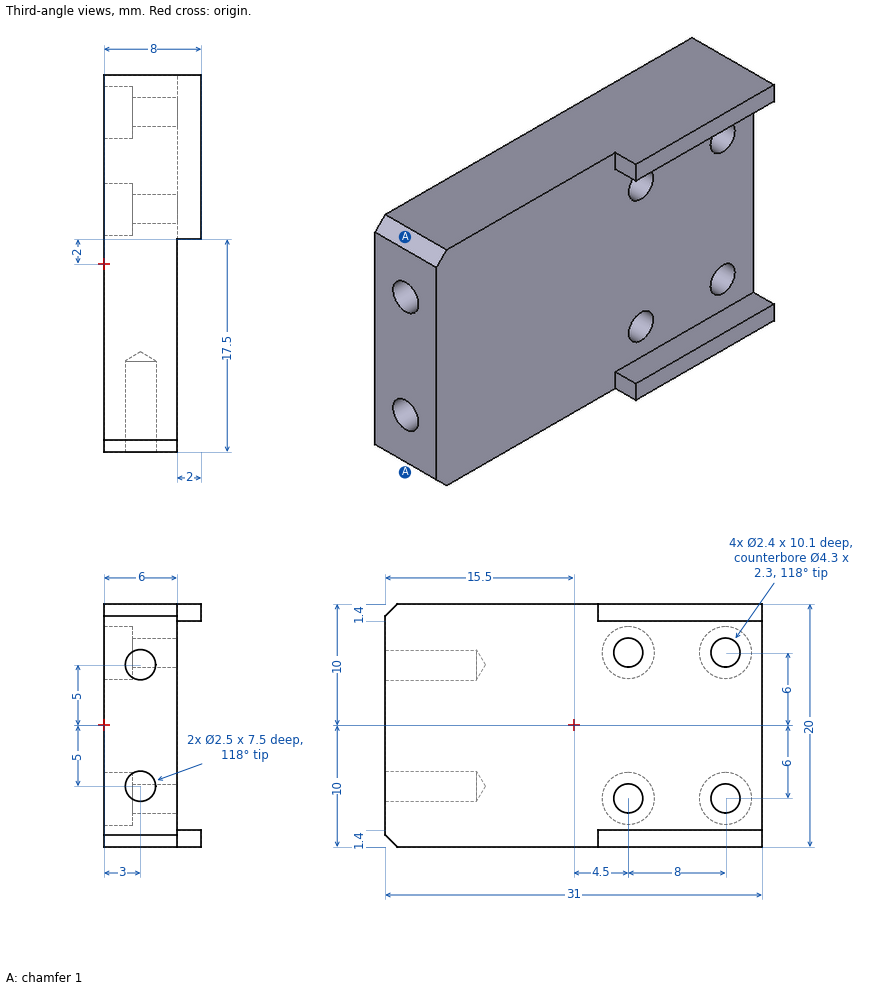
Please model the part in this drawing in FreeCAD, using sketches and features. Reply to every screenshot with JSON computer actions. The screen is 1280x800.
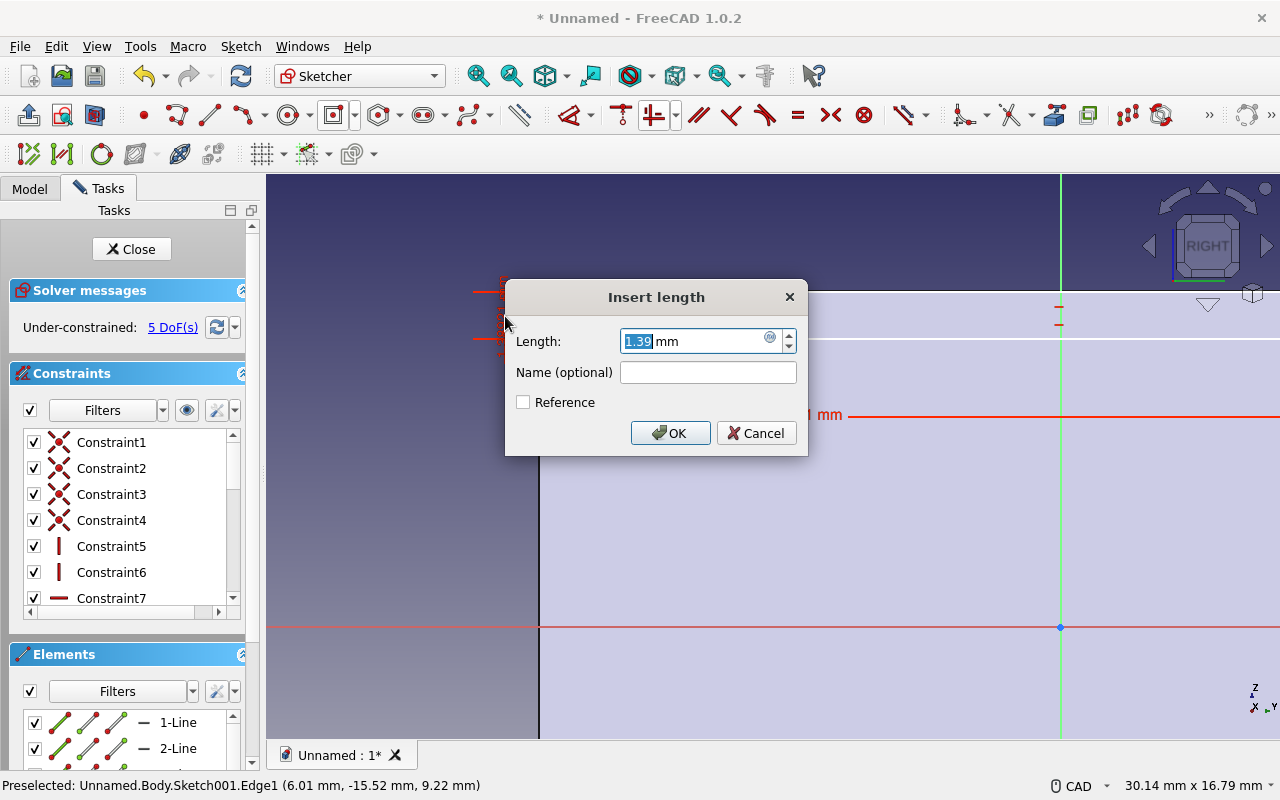
{"action": "type", "text": "1.4"}
{"action": "key", "text": "Return"}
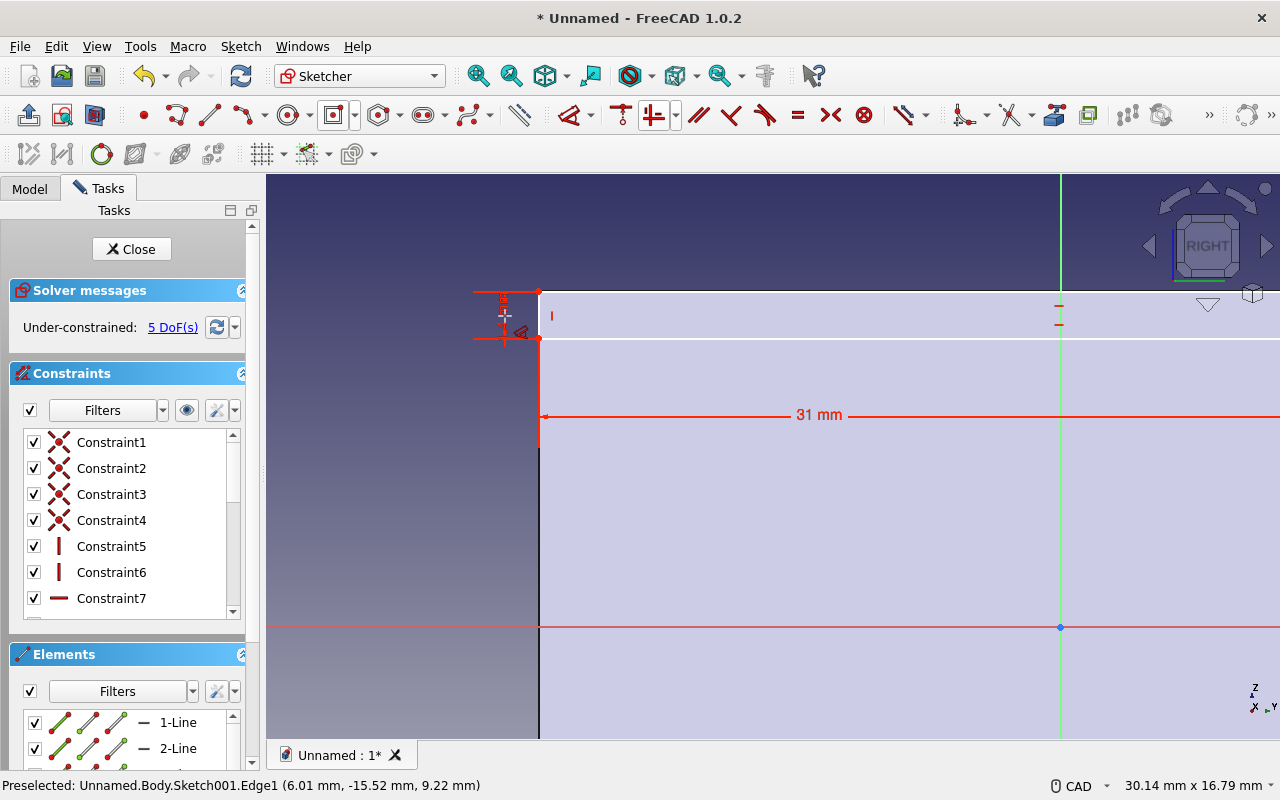
{"action": "scroll", "coordinate": [294, 249], "scroll_direction": "down", "scroll_amount": 3}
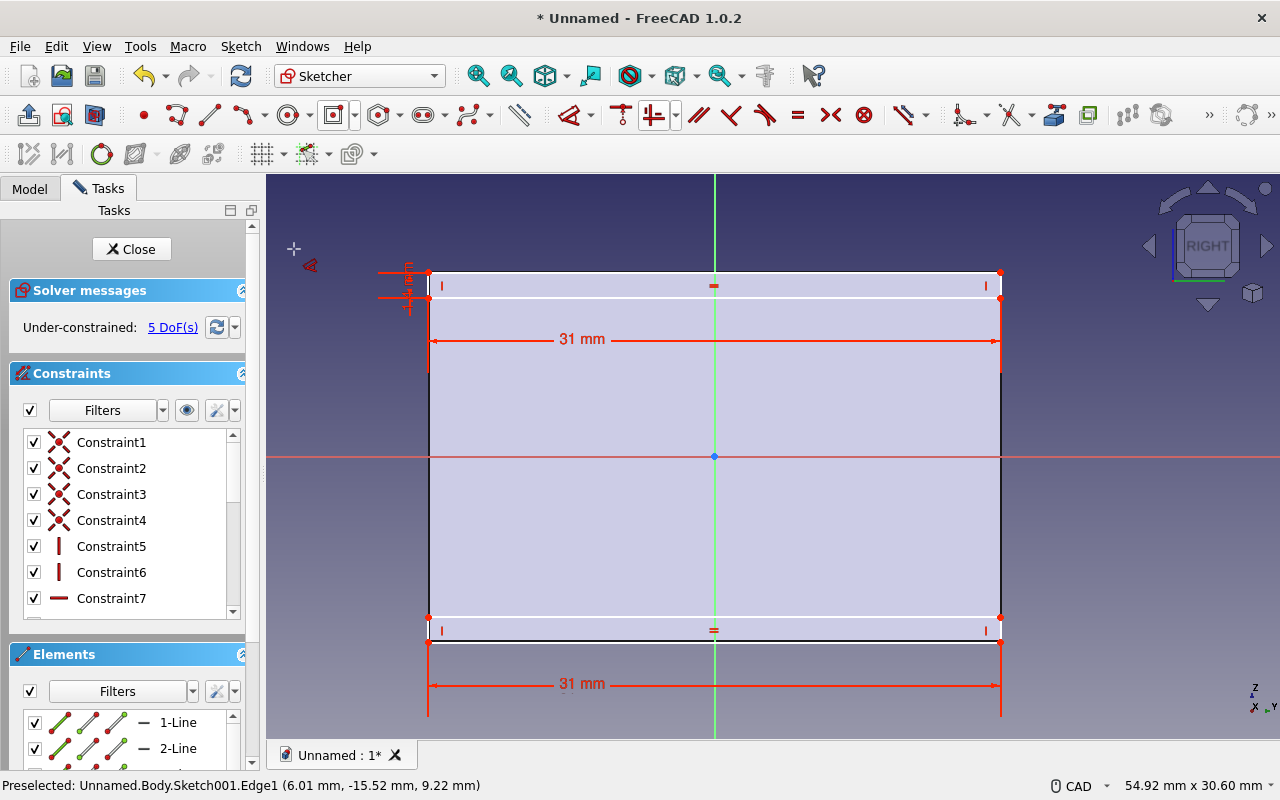
{"action": "scroll", "coordinate": [428, 625], "scroll_direction": "up", "scroll_amount": 3}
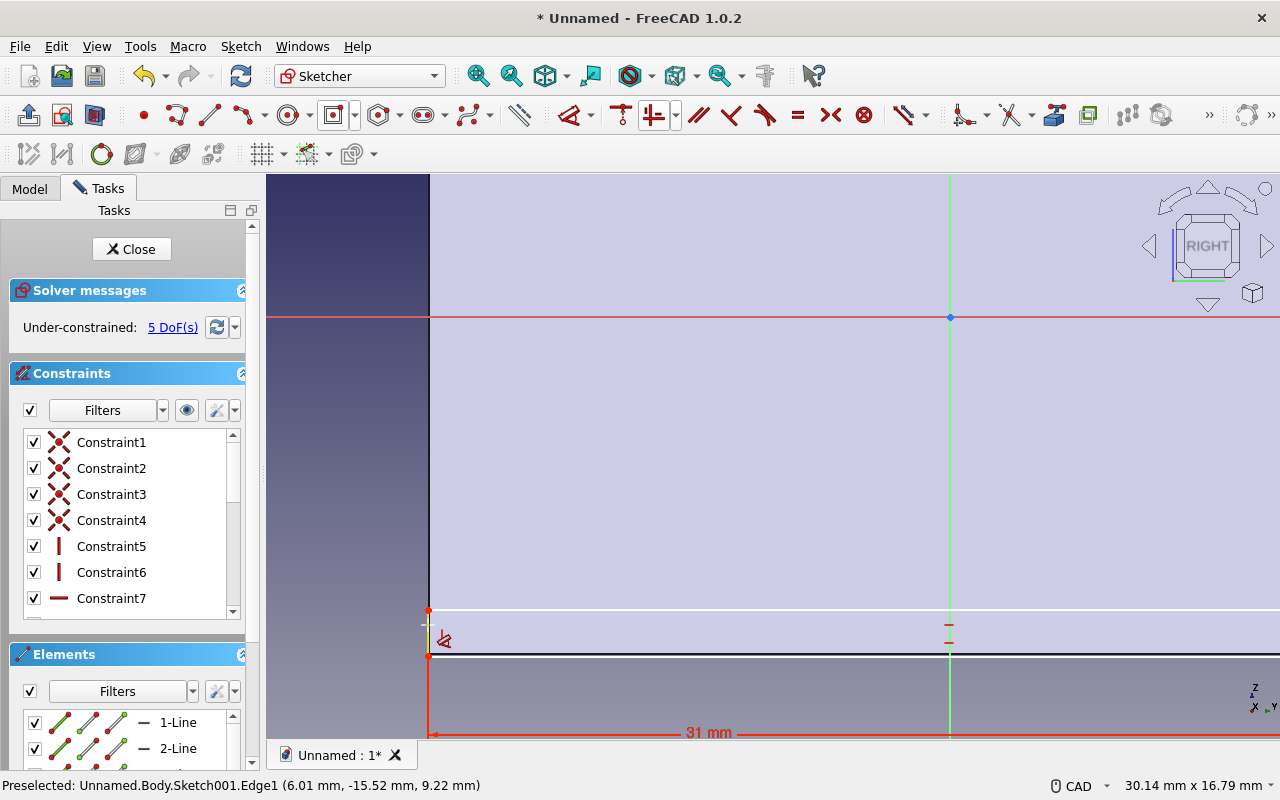
{"action": "left_click", "coordinate": [428, 624]}
{"action": "left_click", "coordinate": [394, 634]}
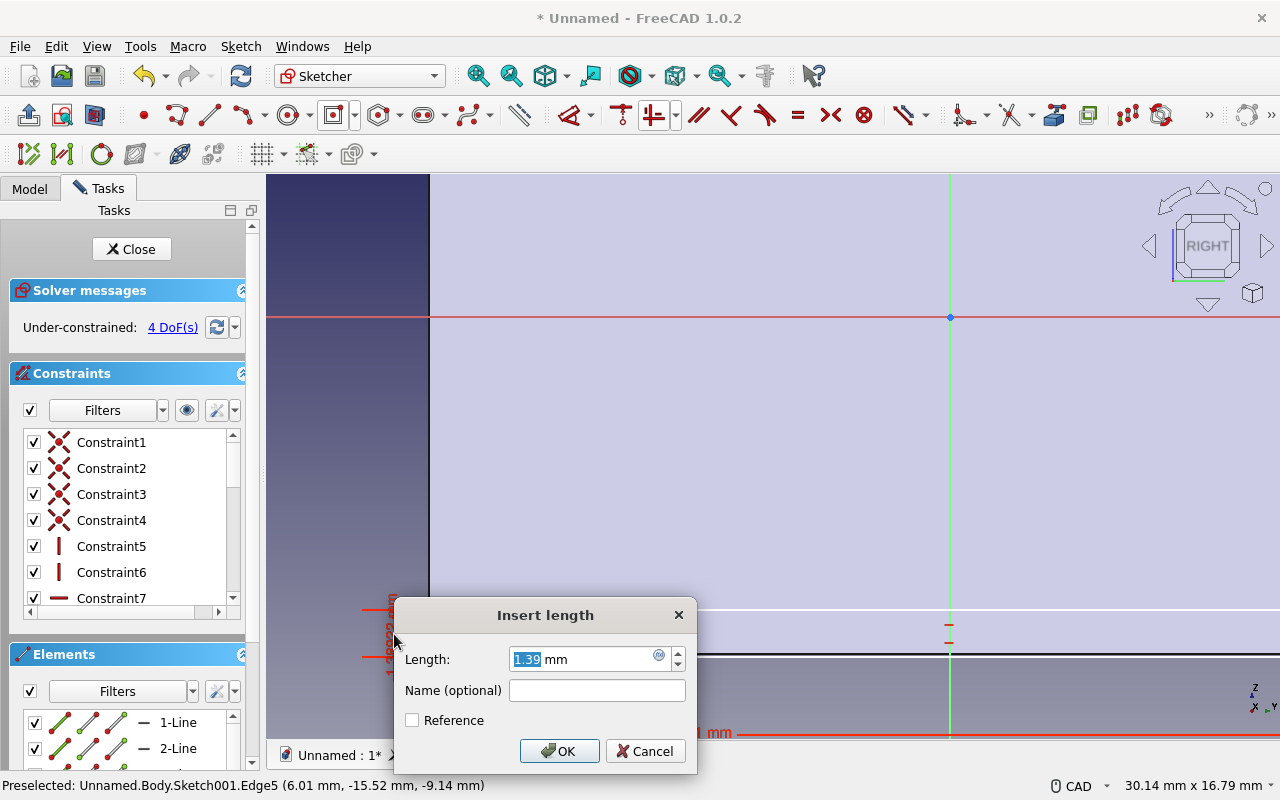
{"action": "type", "text": "1.4"}
{"action": "key", "text": "Return"}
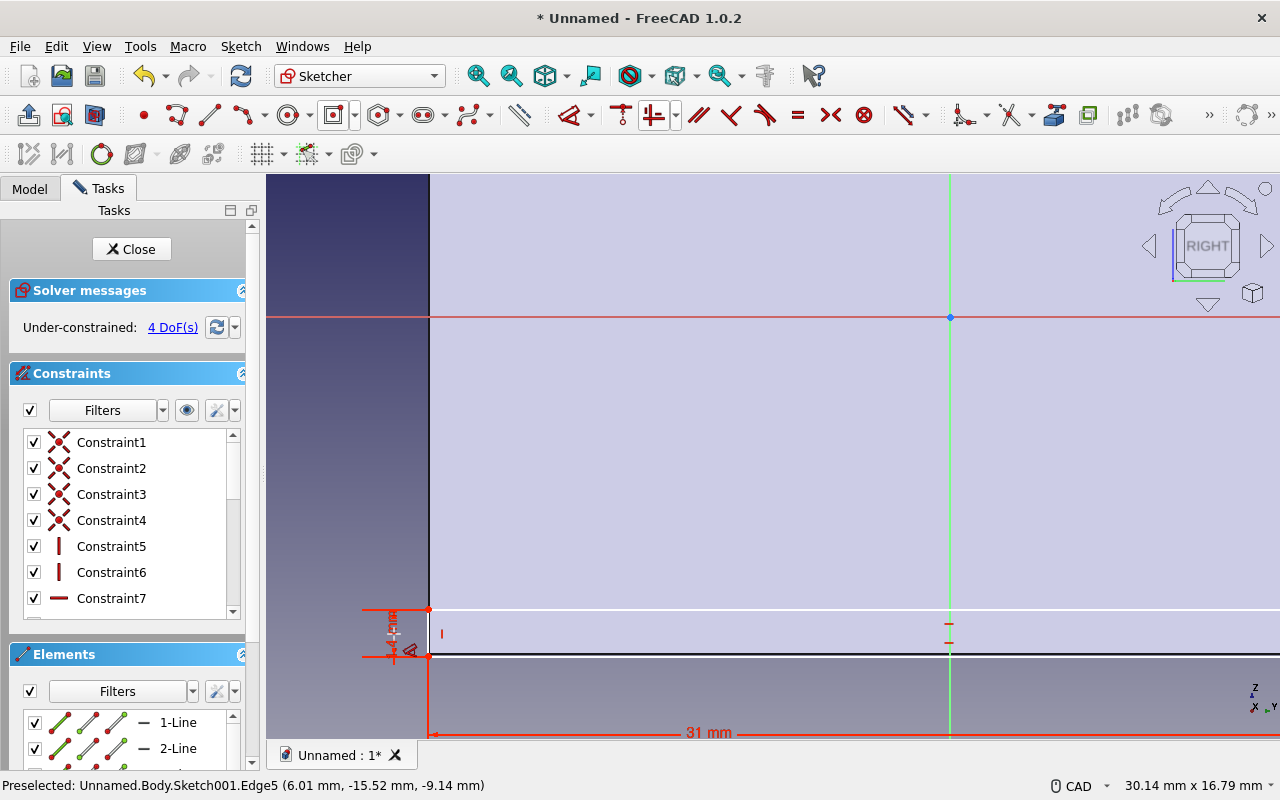
{"action": "scroll", "coordinate": [405, 626], "scroll_direction": "down", "scroll_amount": 3}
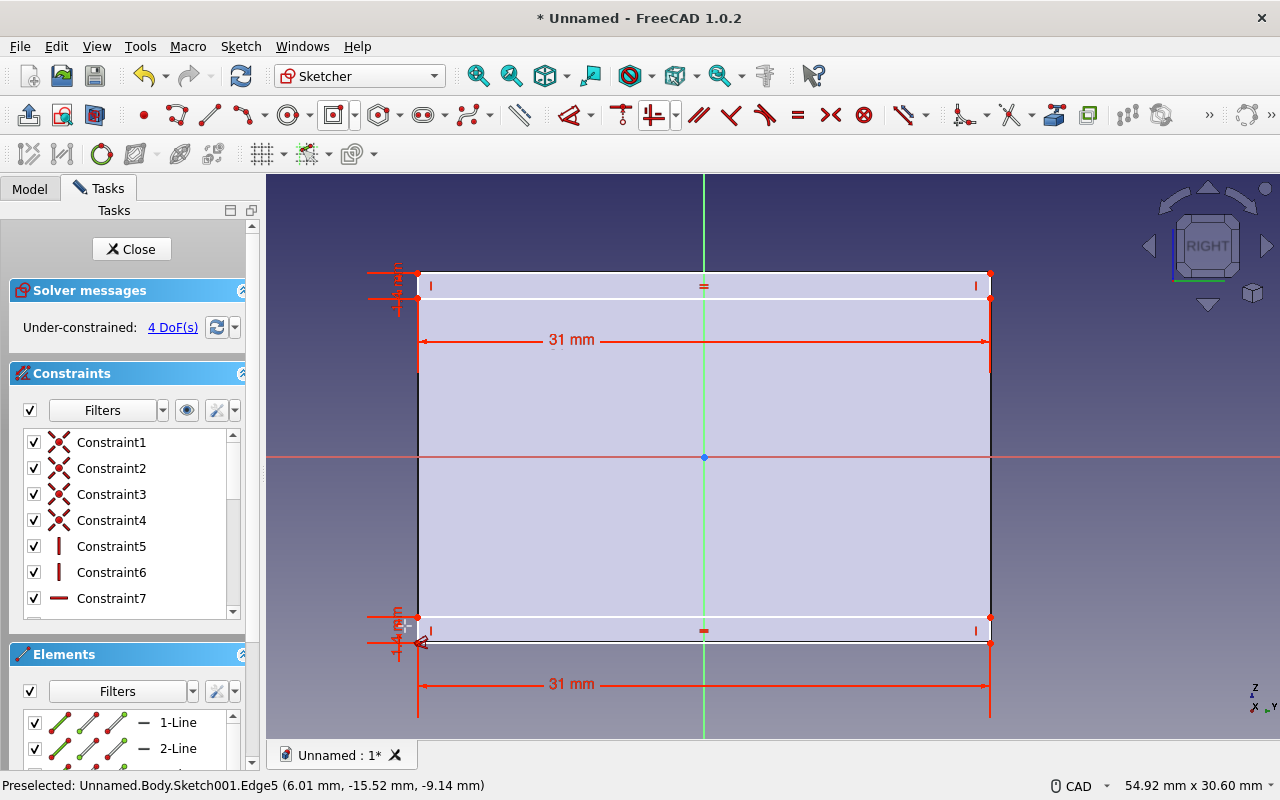
{"action": "left_click", "coordinate": [418, 273]}
{"action": "left_click", "coordinate": [384, 365]}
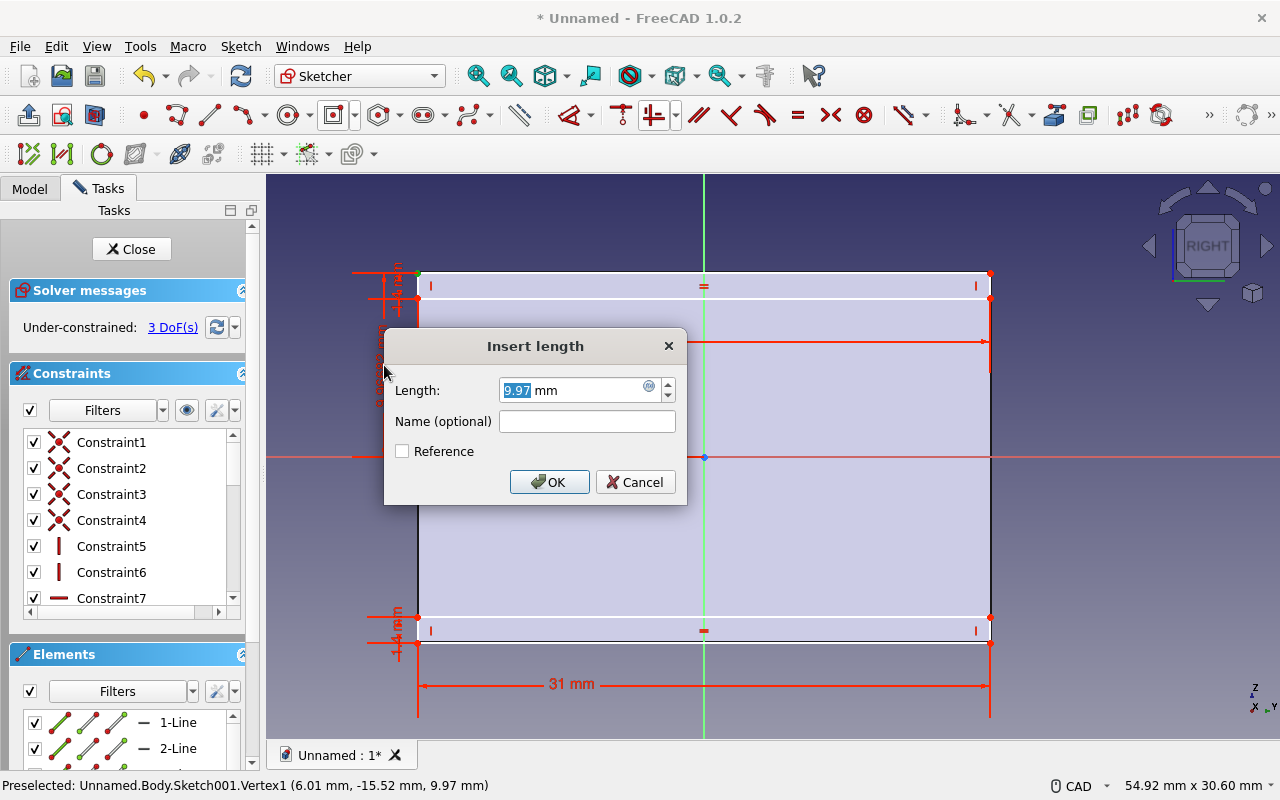
{"action": "type", "text": "10"}
{"action": "key", "text": "Return"}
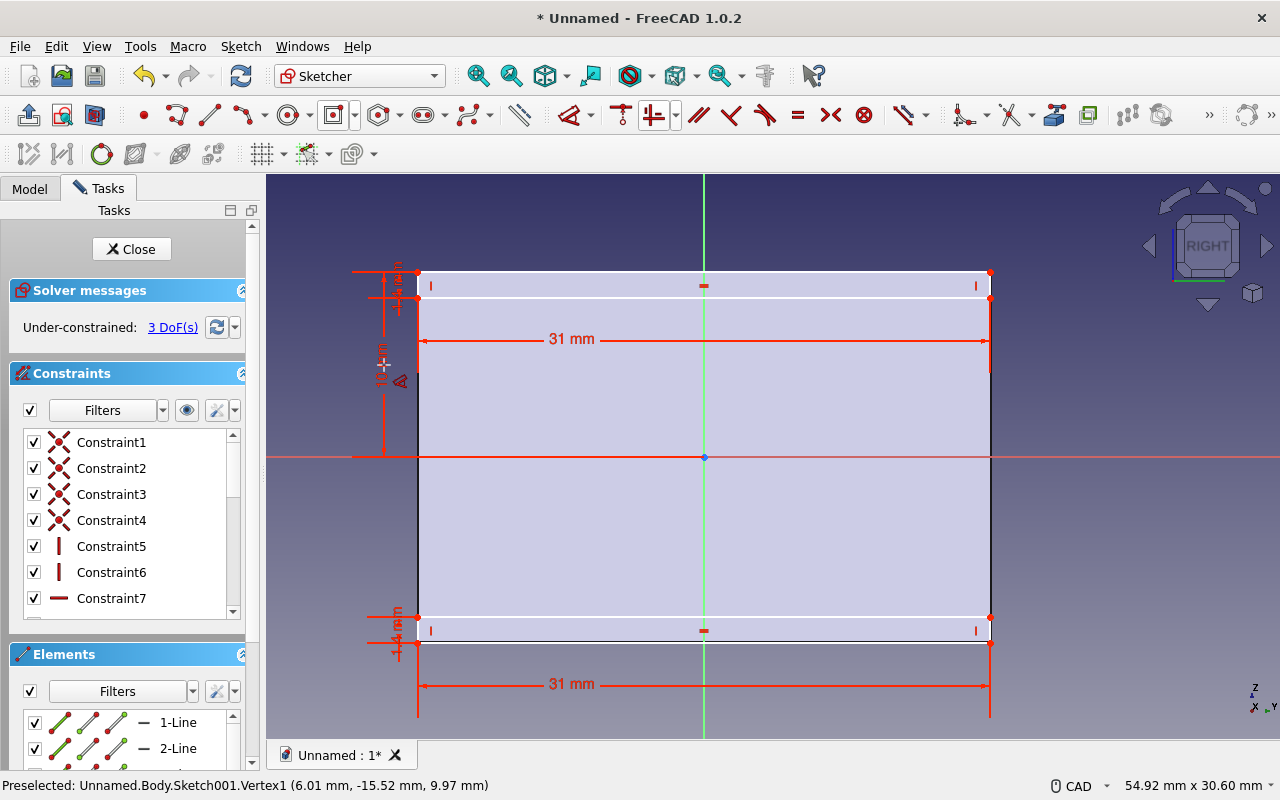
{"action": "left_click", "coordinate": [418, 643]}
{"action": "left_click", "coordinate": [384, 550]}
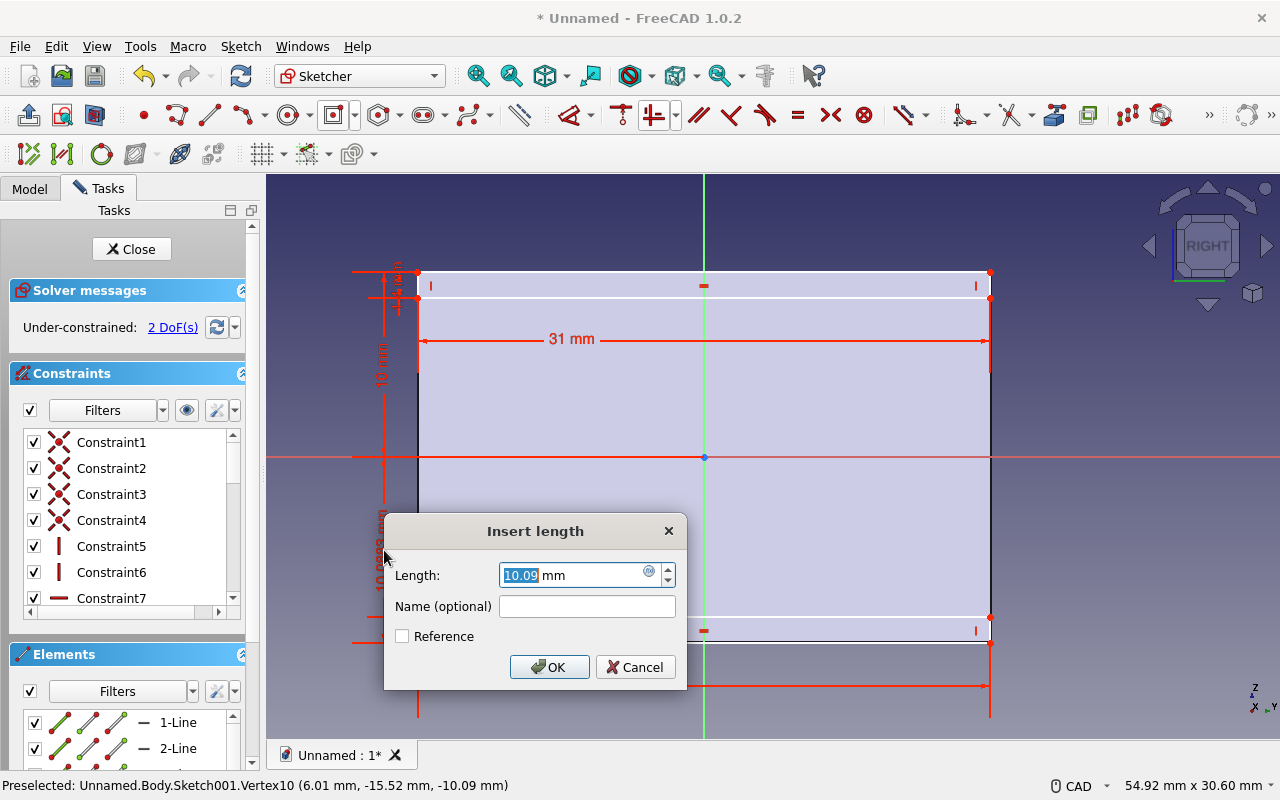
{"action": "type", "text": "10"}
{"action": "key", "text": "Return"}